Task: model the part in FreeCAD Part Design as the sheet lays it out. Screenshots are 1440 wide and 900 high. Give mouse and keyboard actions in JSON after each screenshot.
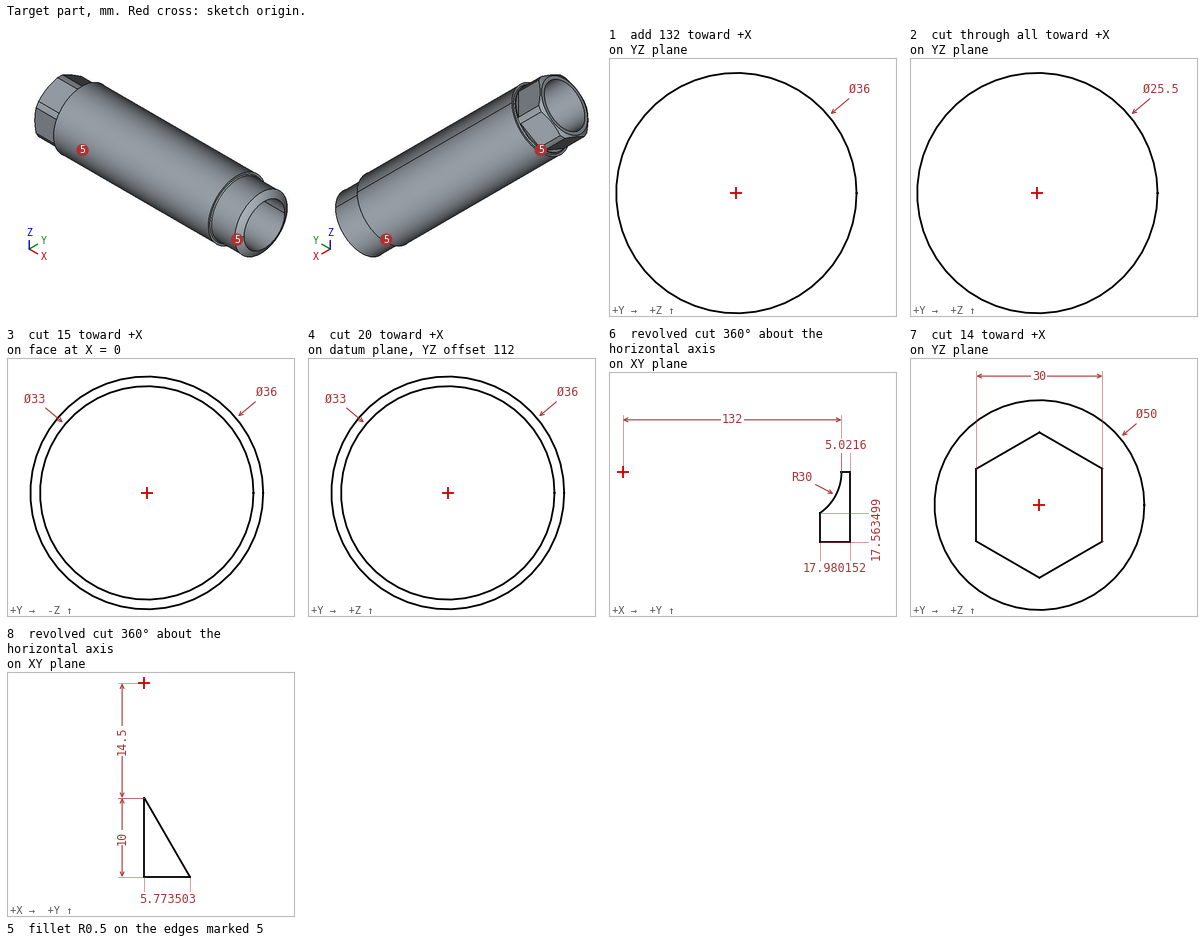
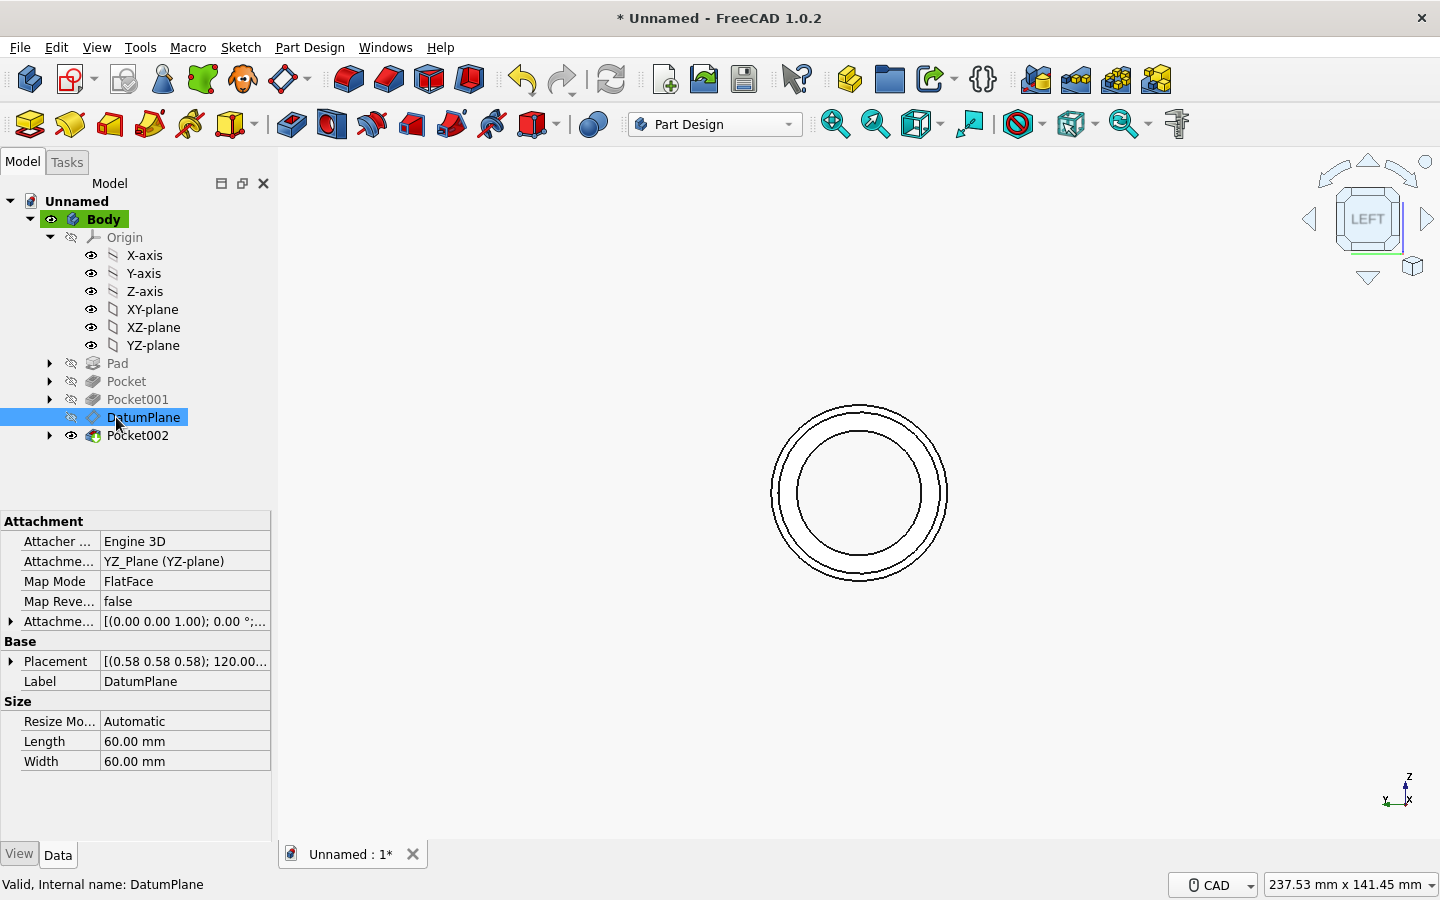
{"action": "key", "text": "v f"}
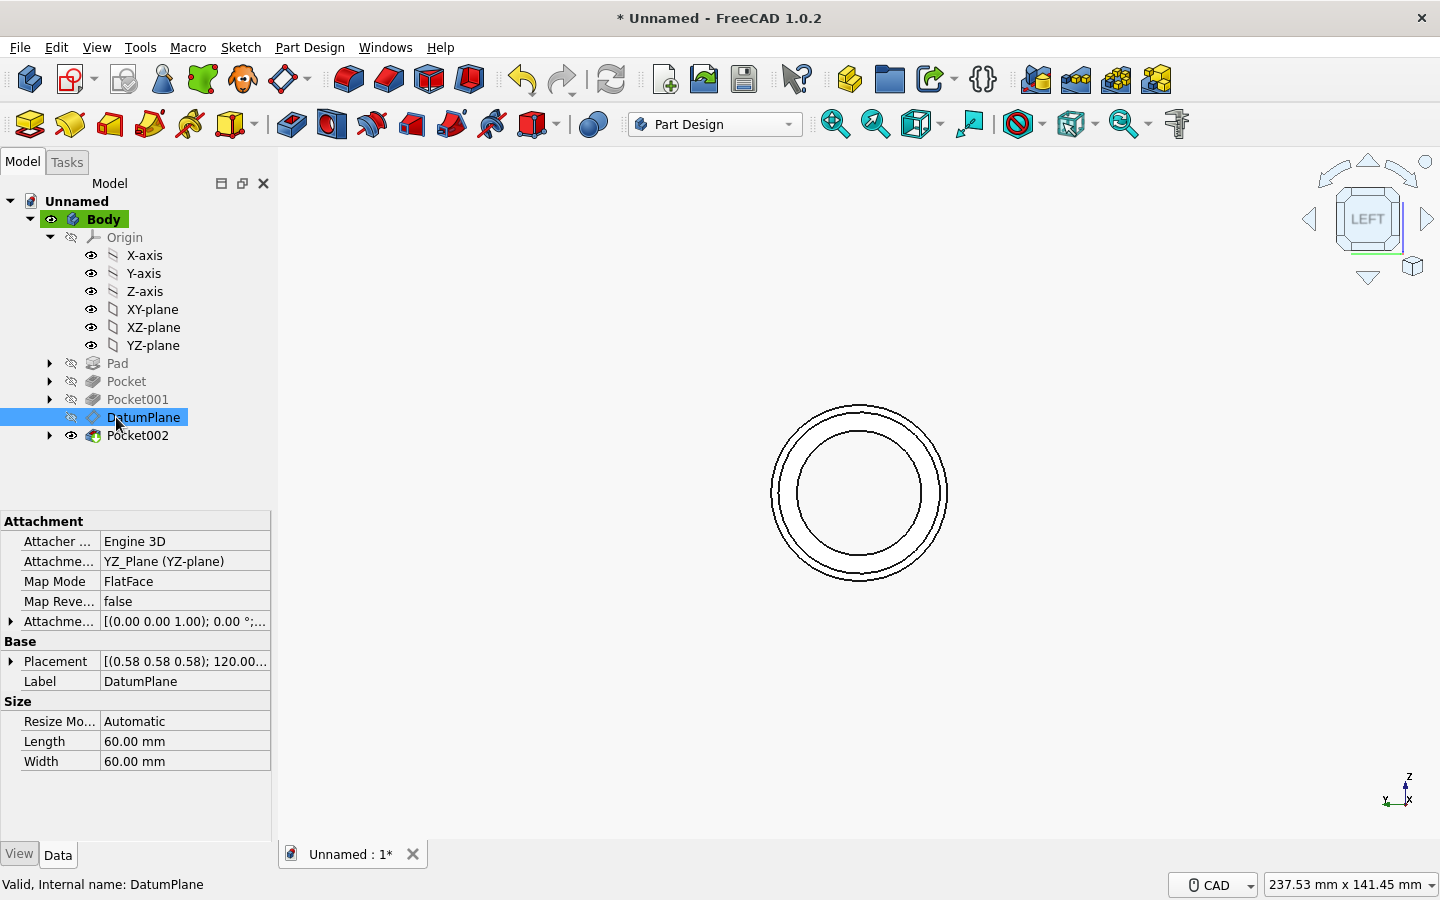
{"action": "key", "text": "0"}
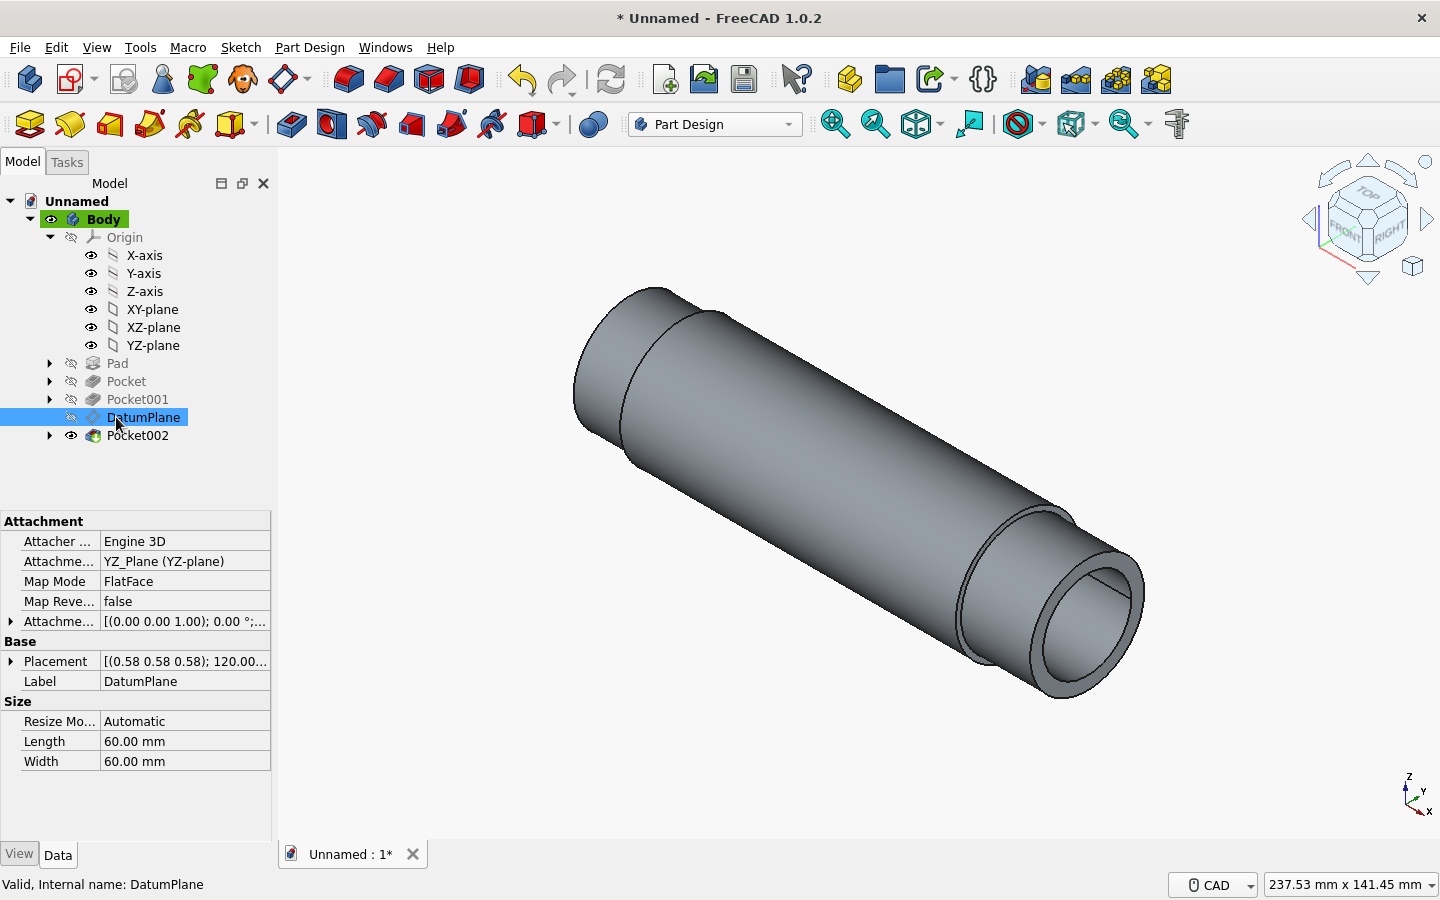
{"action": "key", "text": "2"}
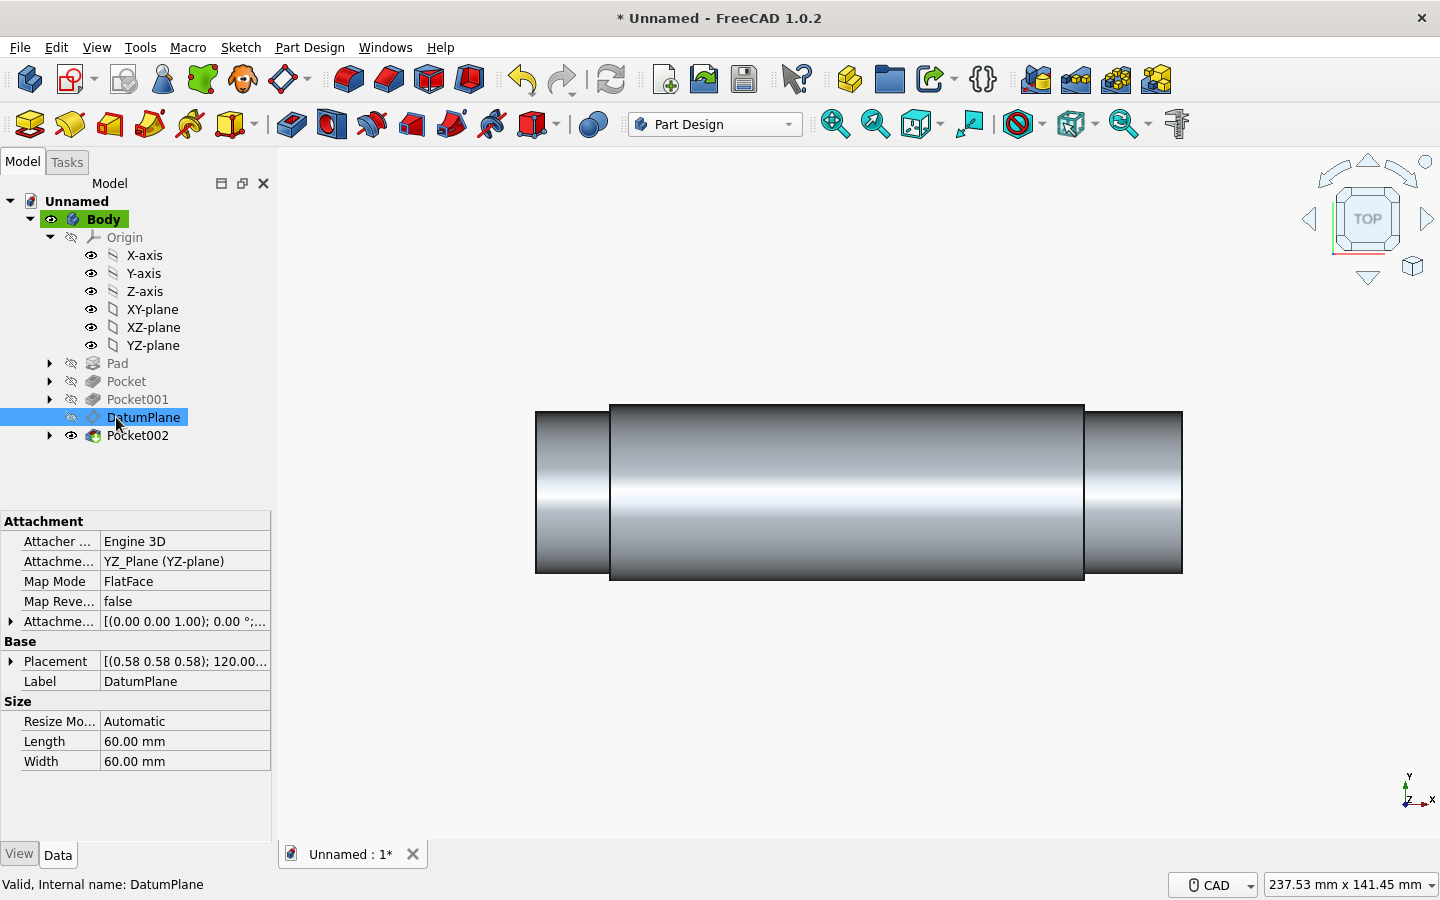
{"action": "key", "text": "1"}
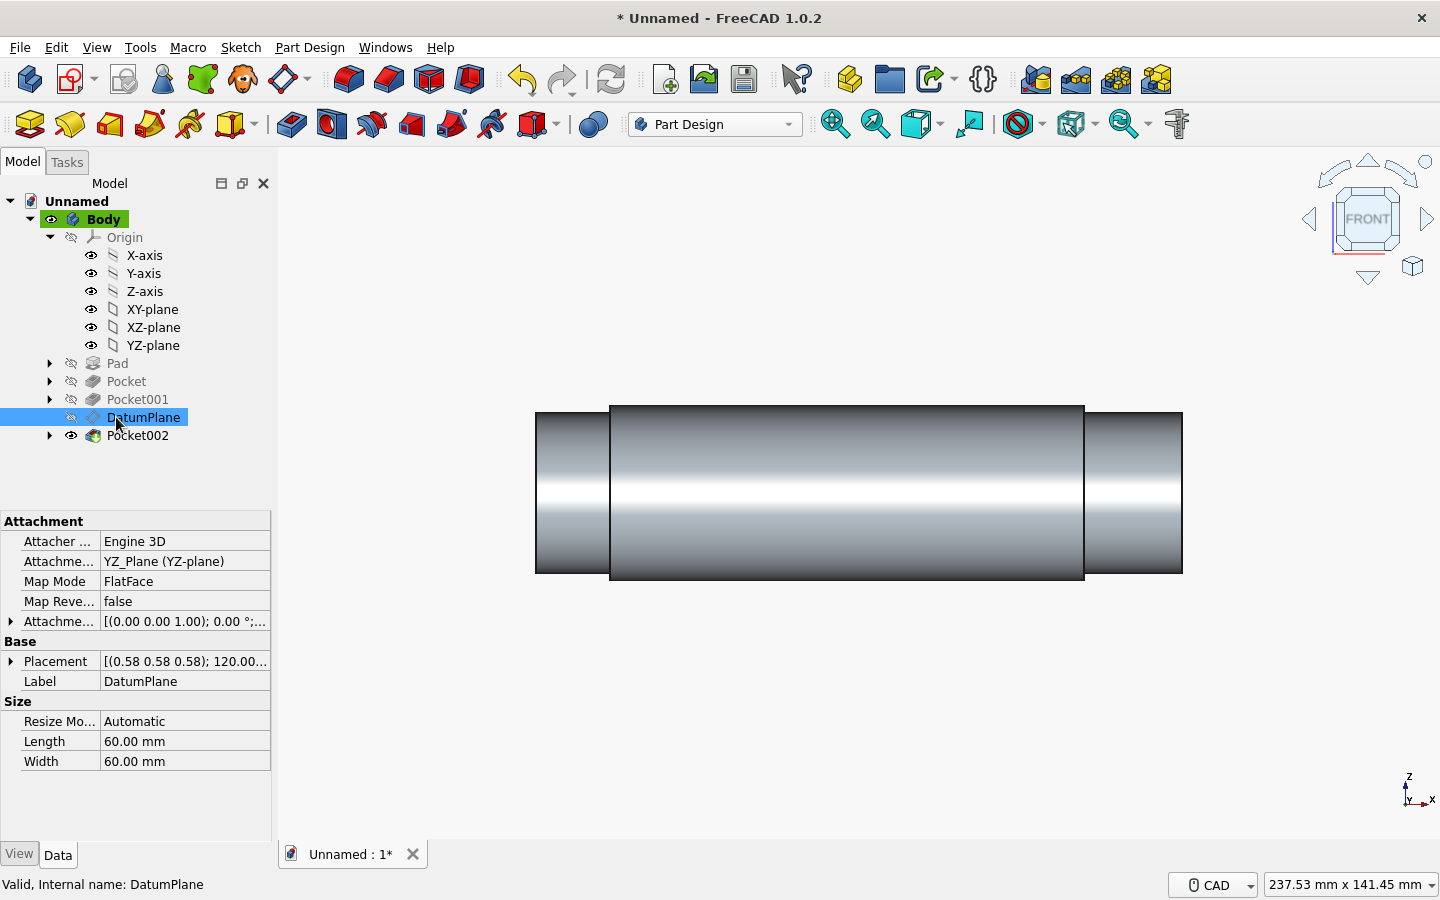
{"action": "key", "text": "3"}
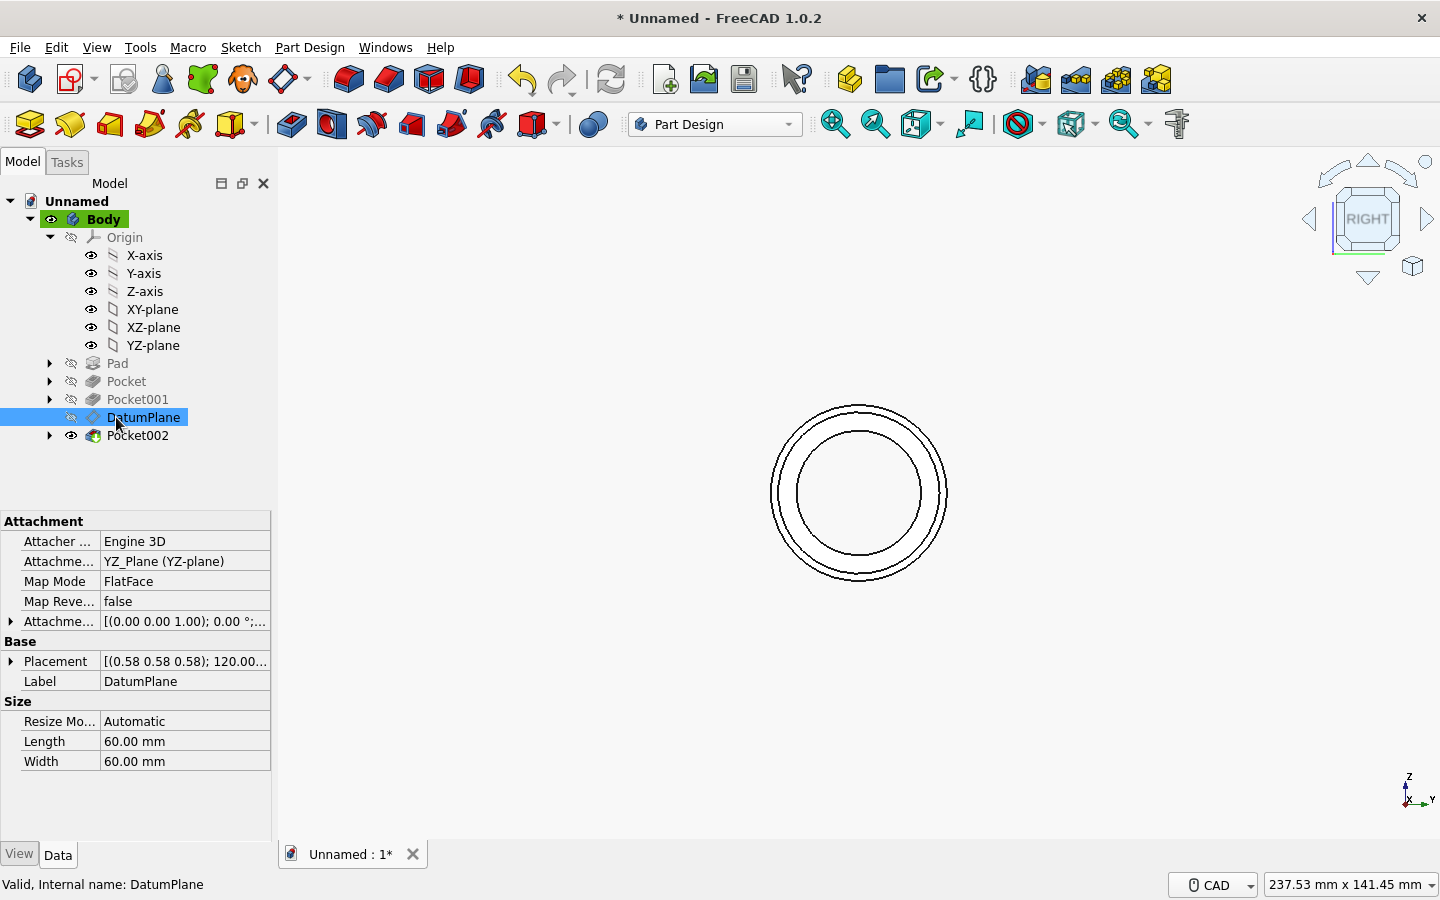
{"action": "left_click", "coordinate": [836, 124]}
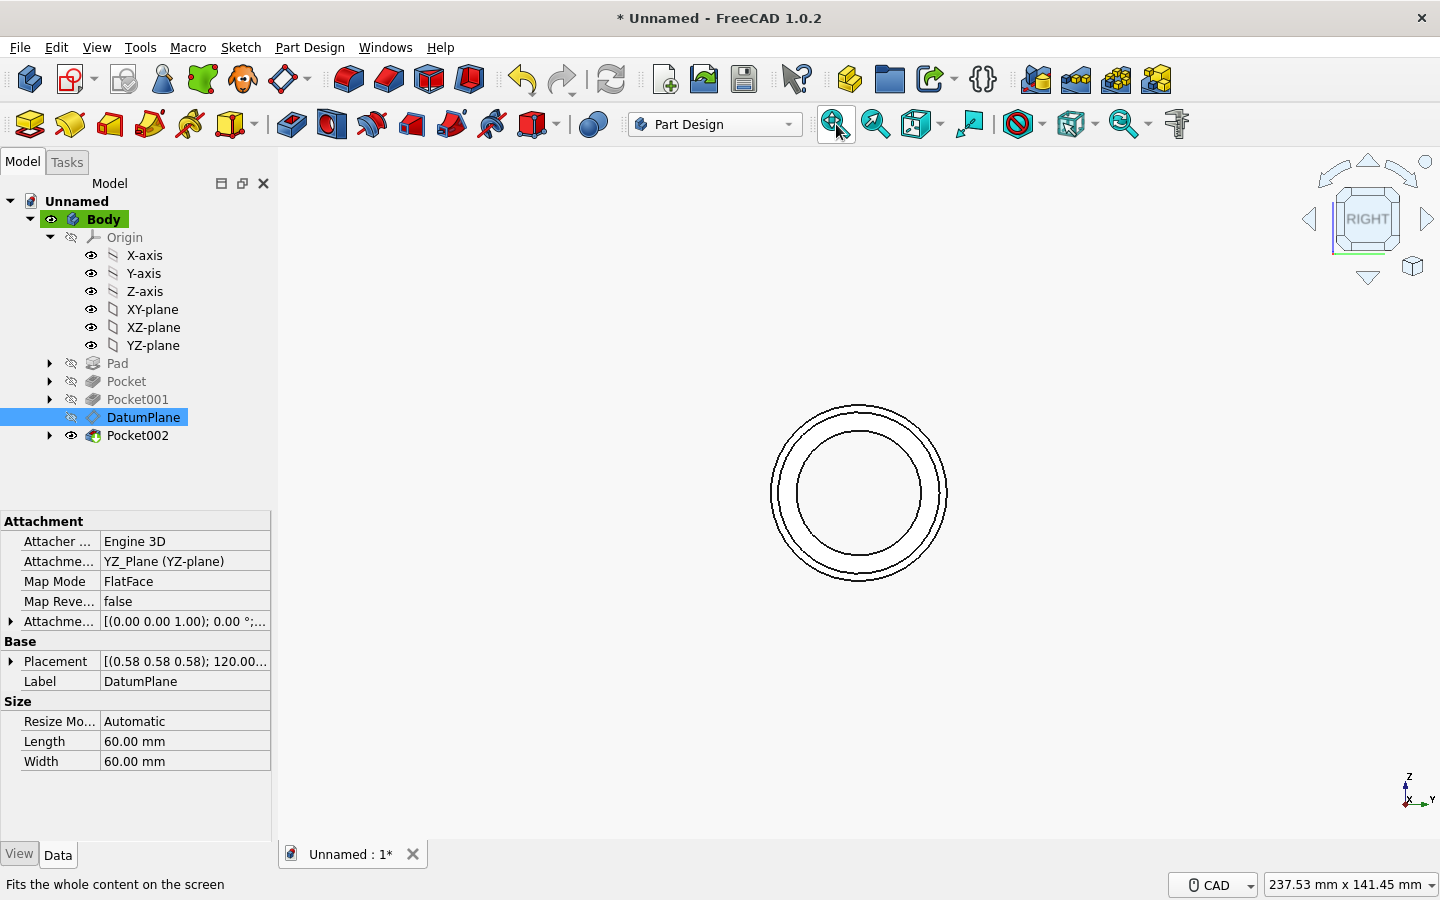
{"action": "key", "text": "5"}